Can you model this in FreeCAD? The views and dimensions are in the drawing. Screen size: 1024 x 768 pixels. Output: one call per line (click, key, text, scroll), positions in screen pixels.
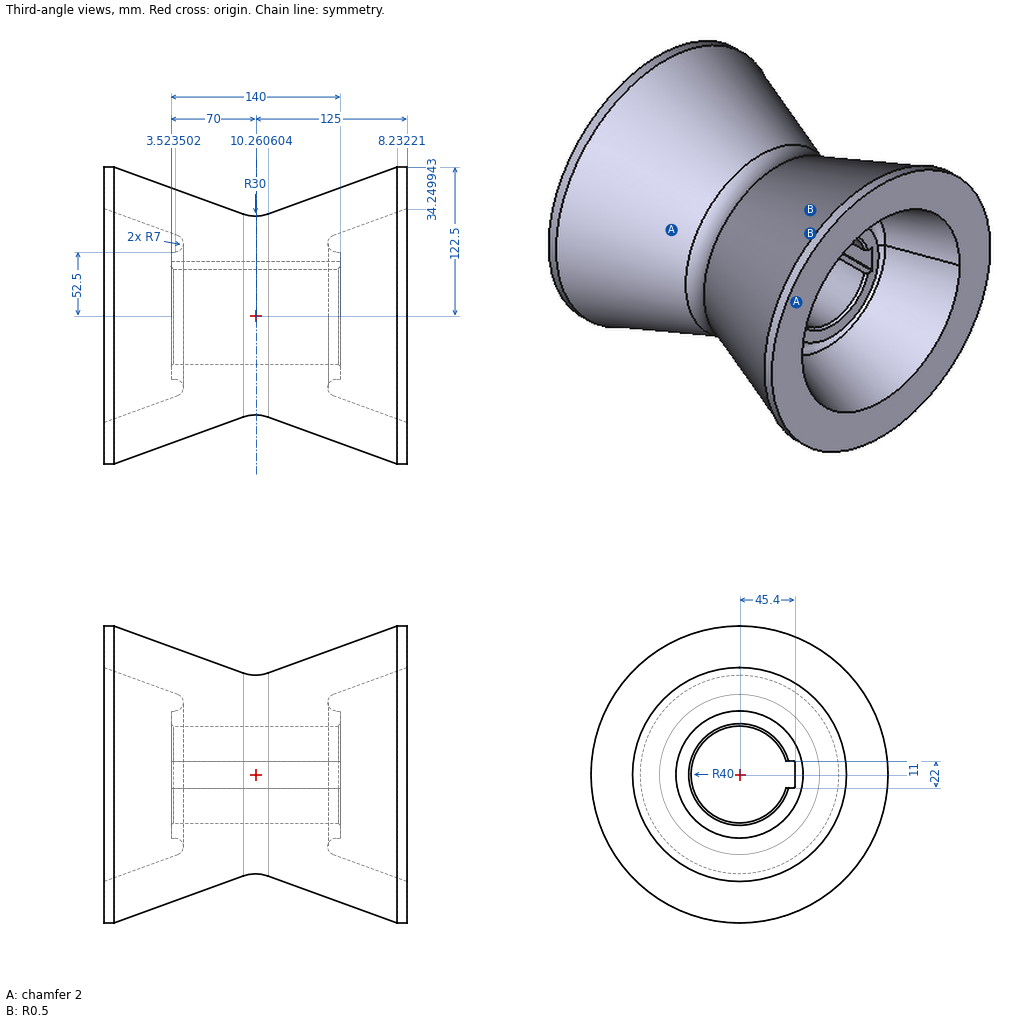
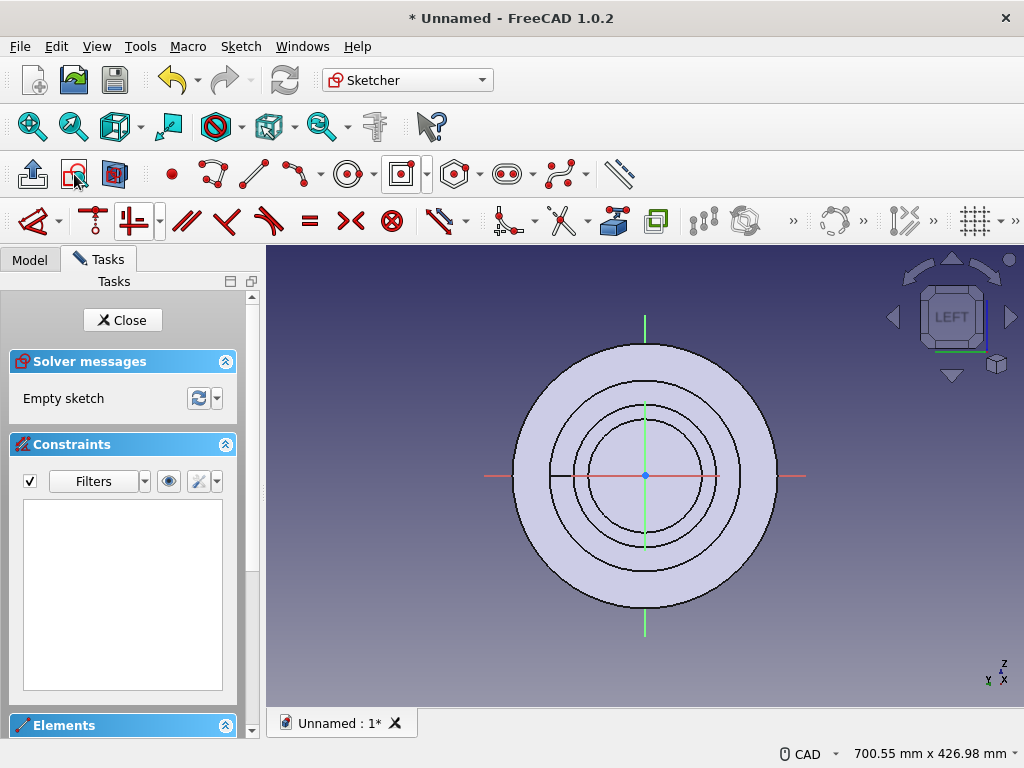
scroll(664, 476, up, 7)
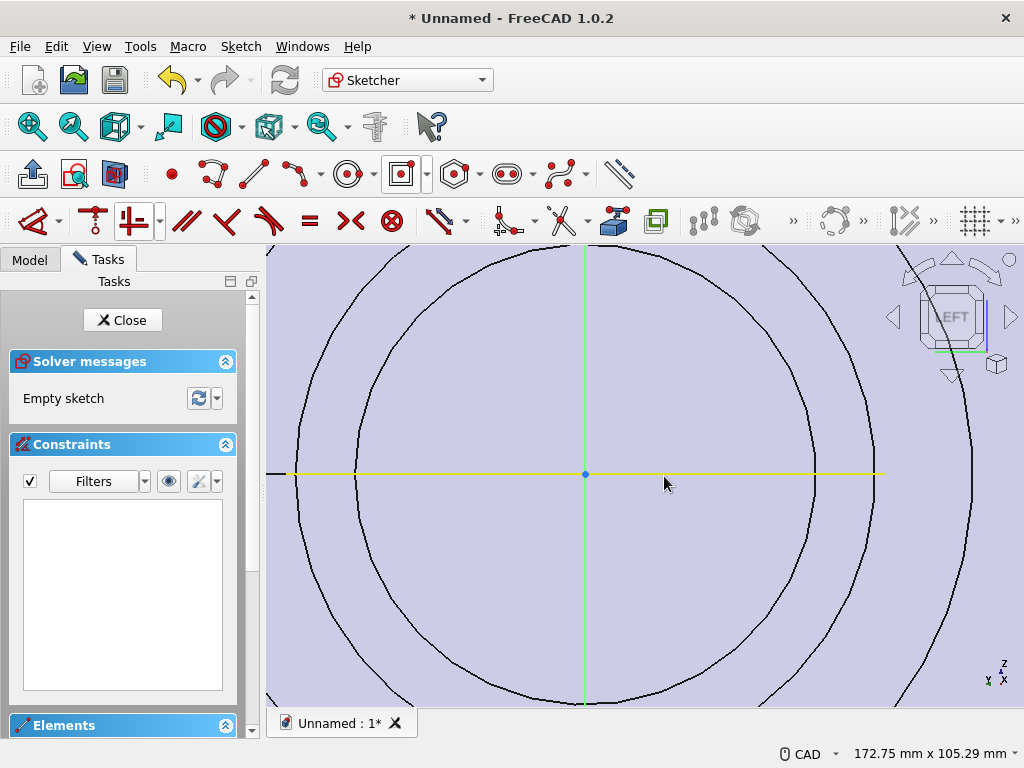
click(213, 174)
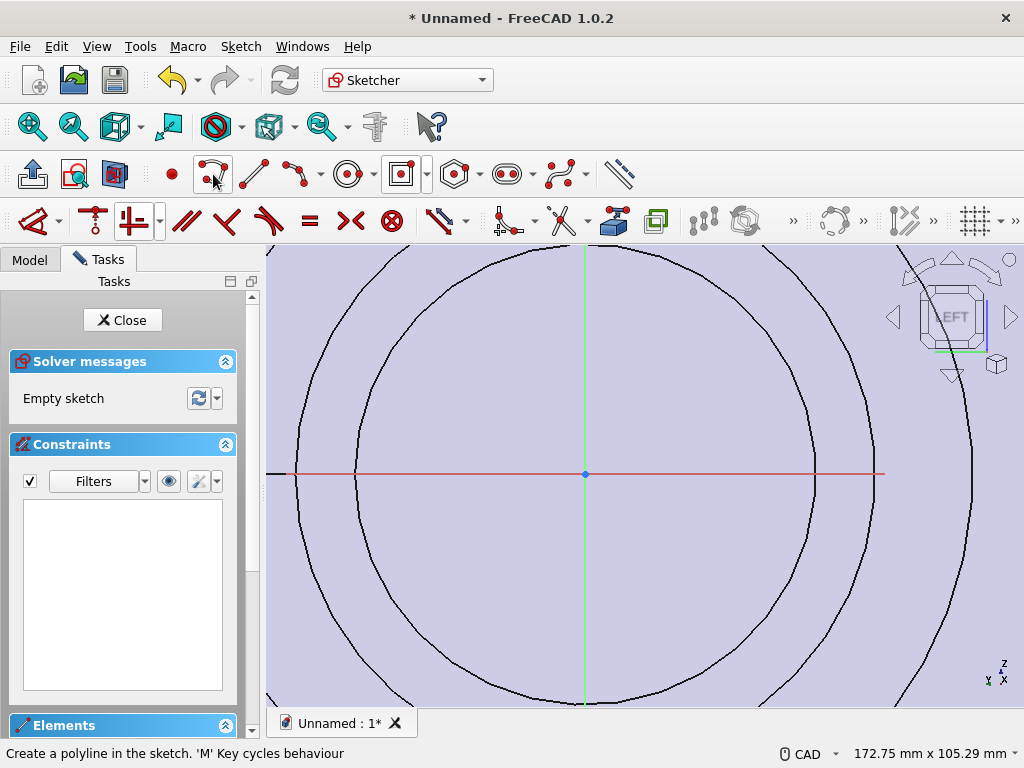
click(417, 426)
click(386, 426)
click(386, 523)
click(417, 523)
right_click(417, 523)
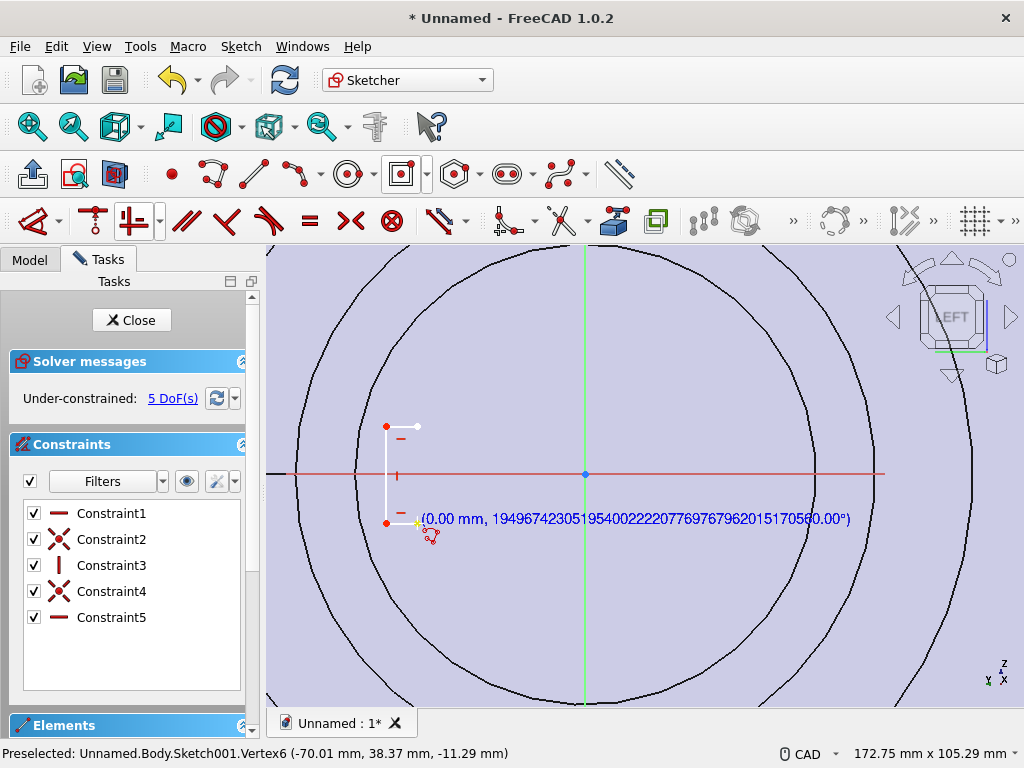
click(294, 174)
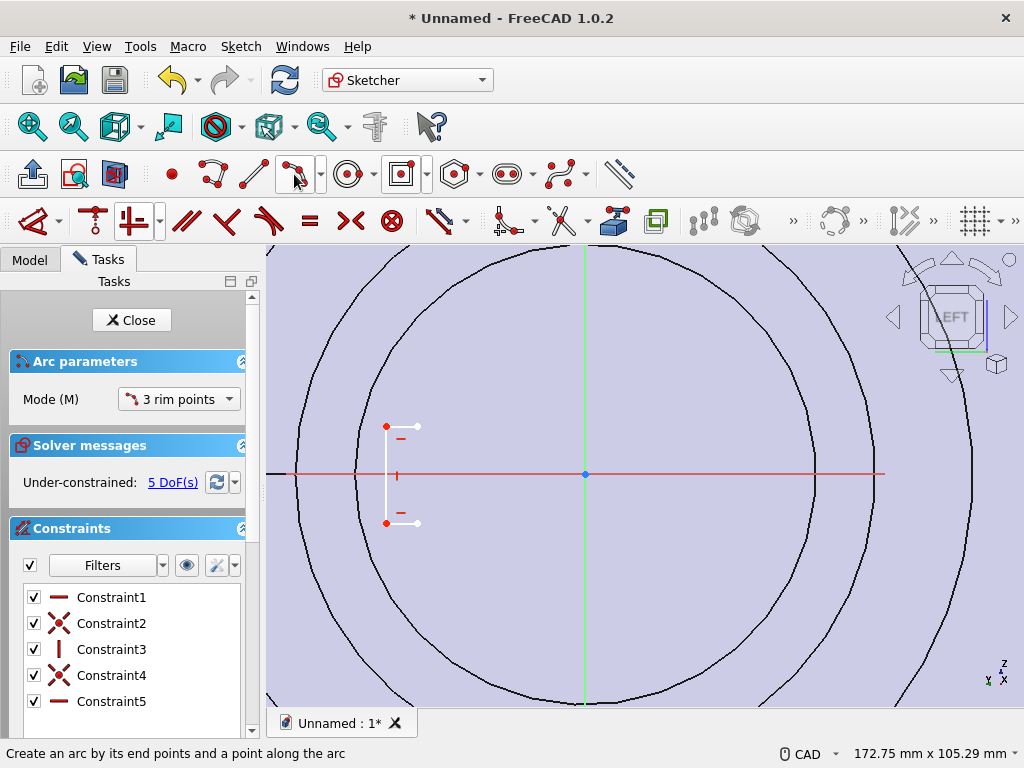
click(417, 524)
click(417, 427)
click(733, 570)
key(Escape)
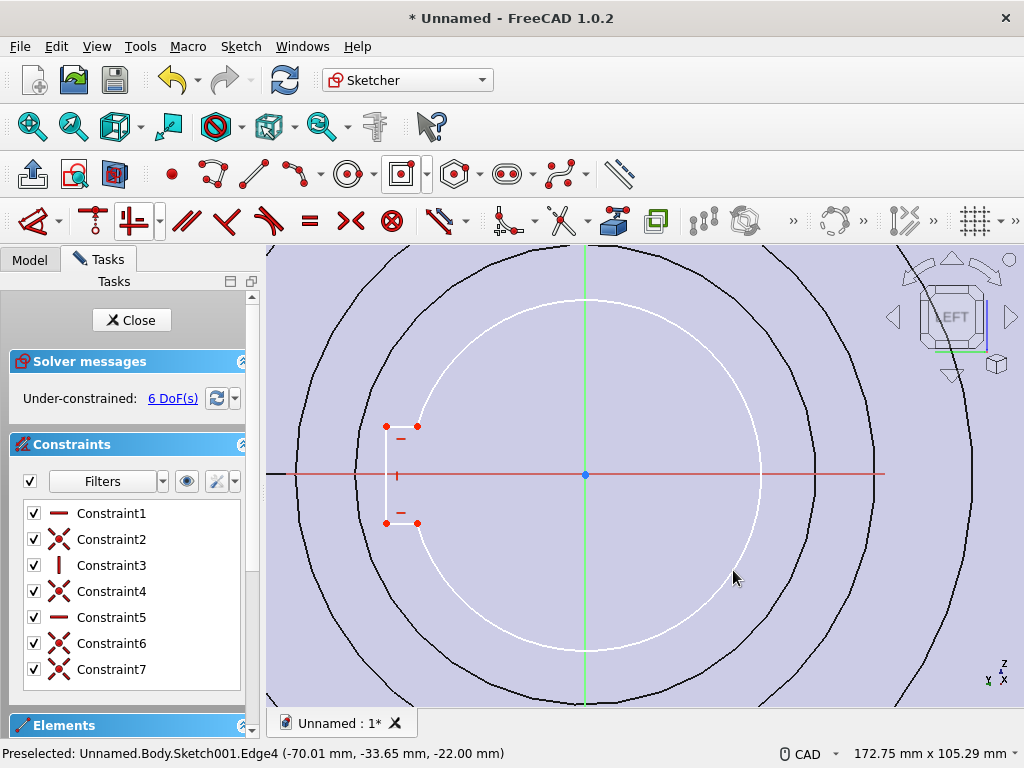
drag(575, 464, 596, 485)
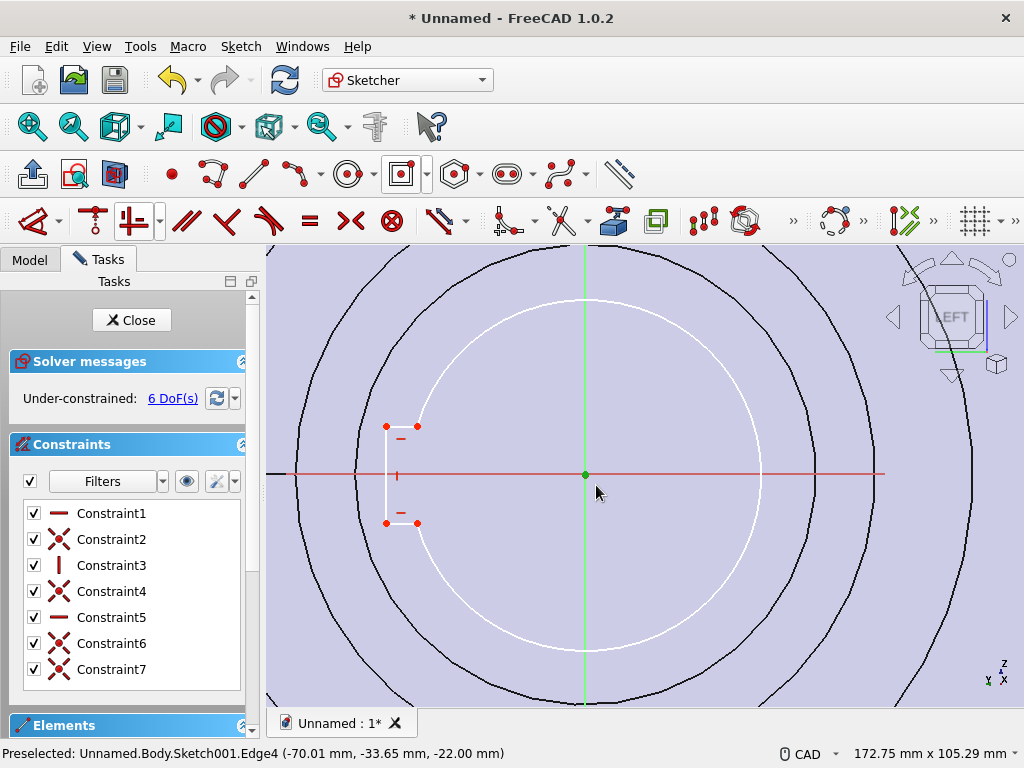
click(93, 222)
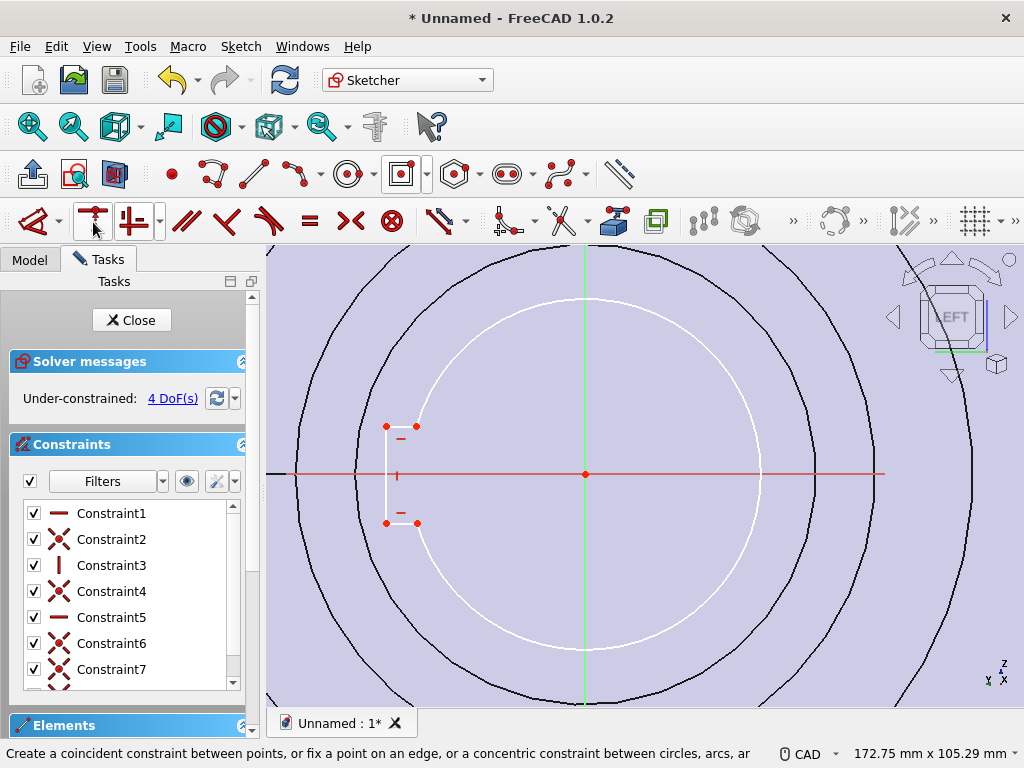
click(32, 222)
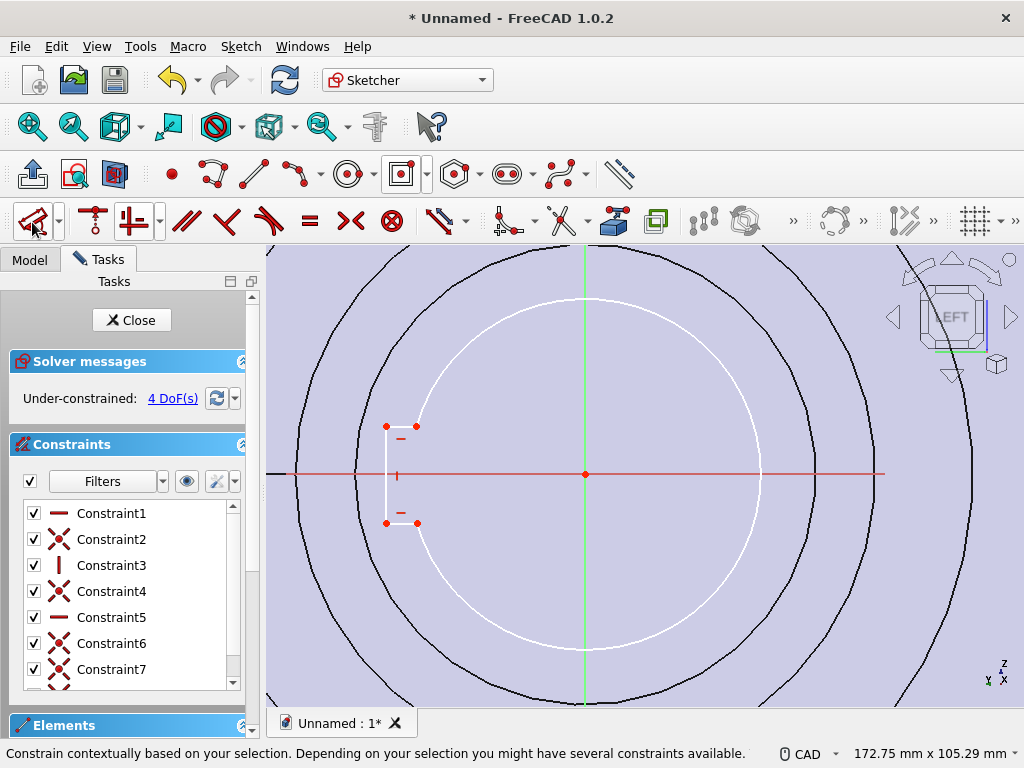
click(659, 634)
click(672, 663)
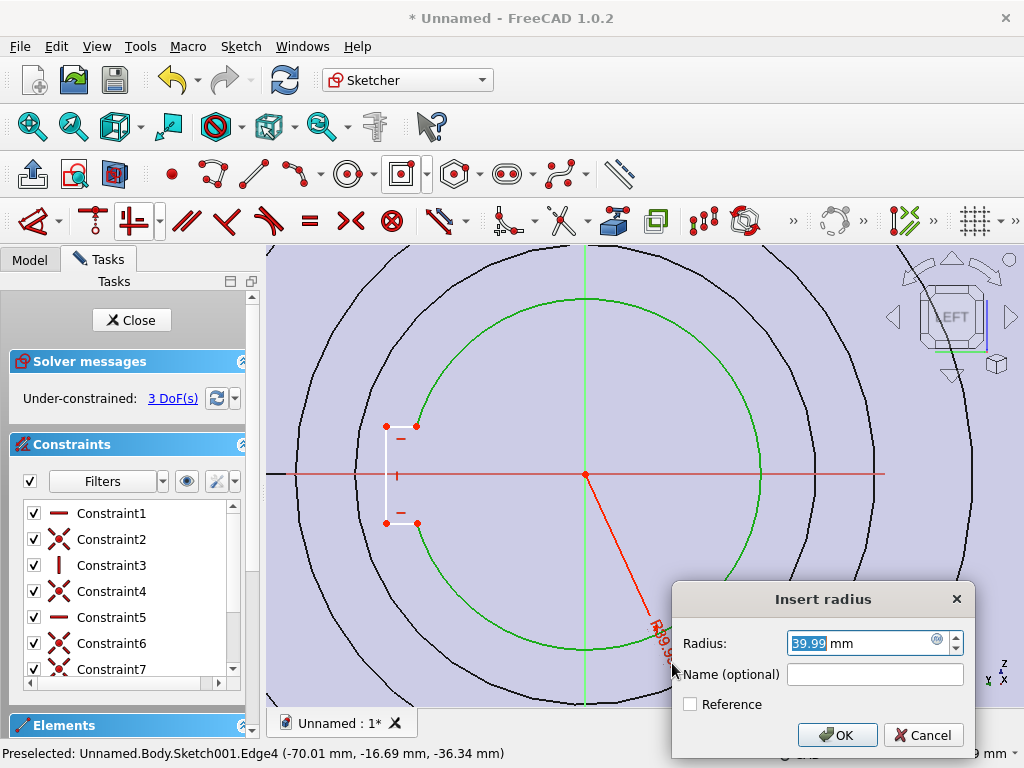
text(40)
key(Return)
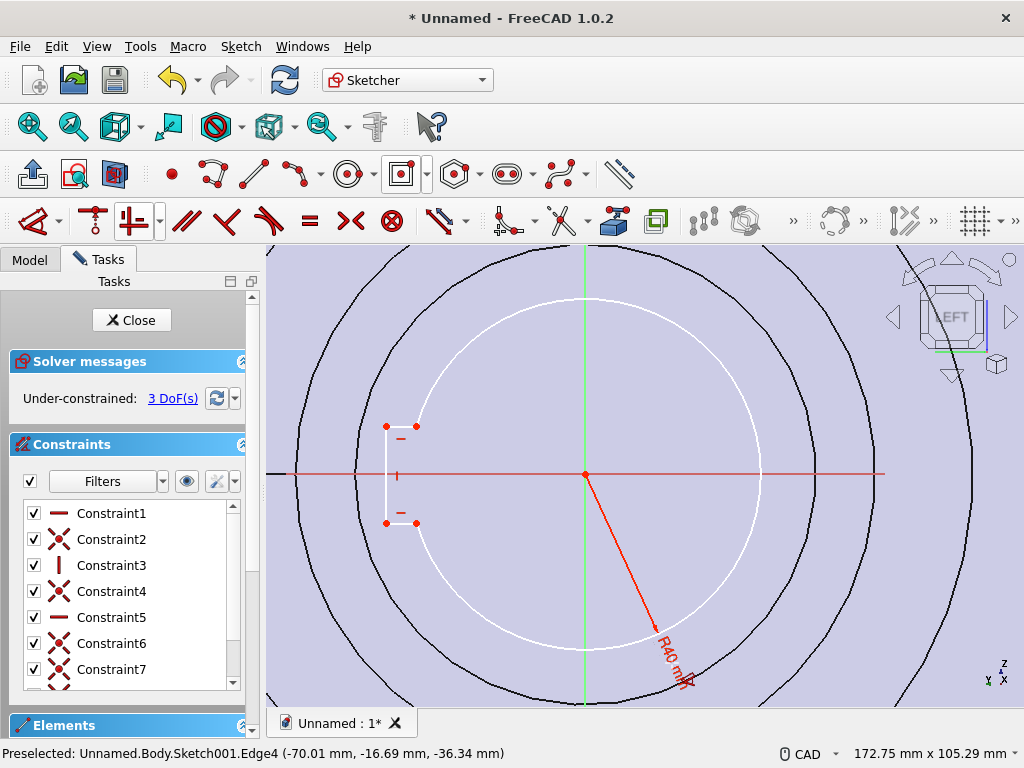
click(386, 456)
click(352, 453)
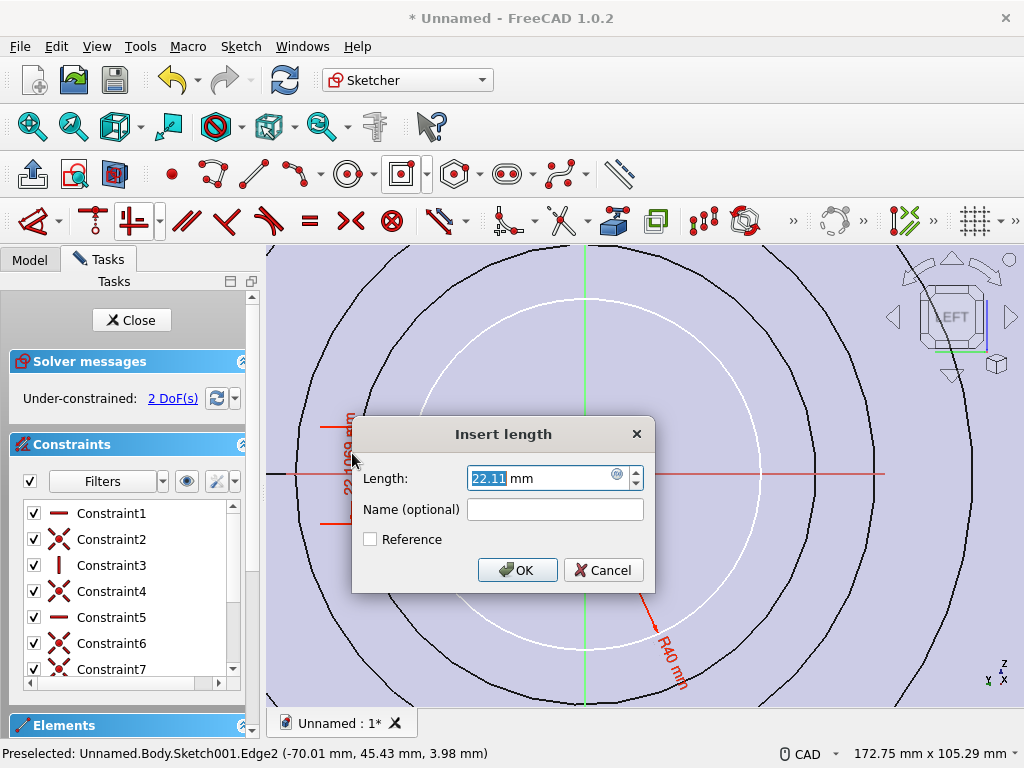
text(22)
key(Return)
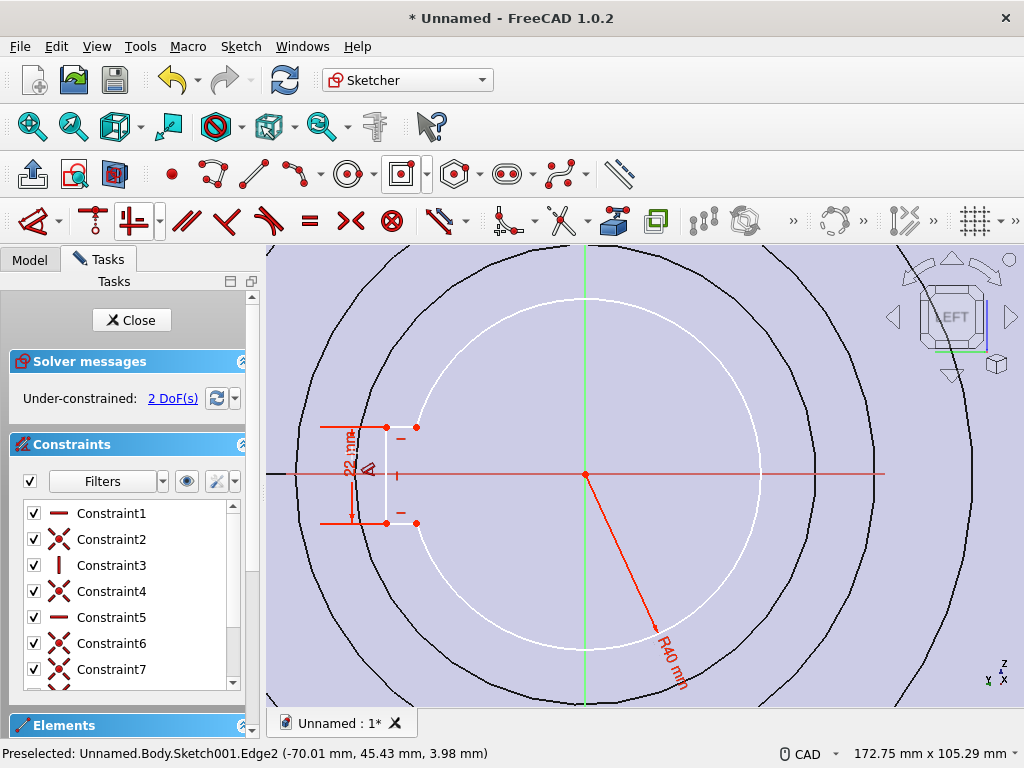
click(416, 427)
click(619, 451)